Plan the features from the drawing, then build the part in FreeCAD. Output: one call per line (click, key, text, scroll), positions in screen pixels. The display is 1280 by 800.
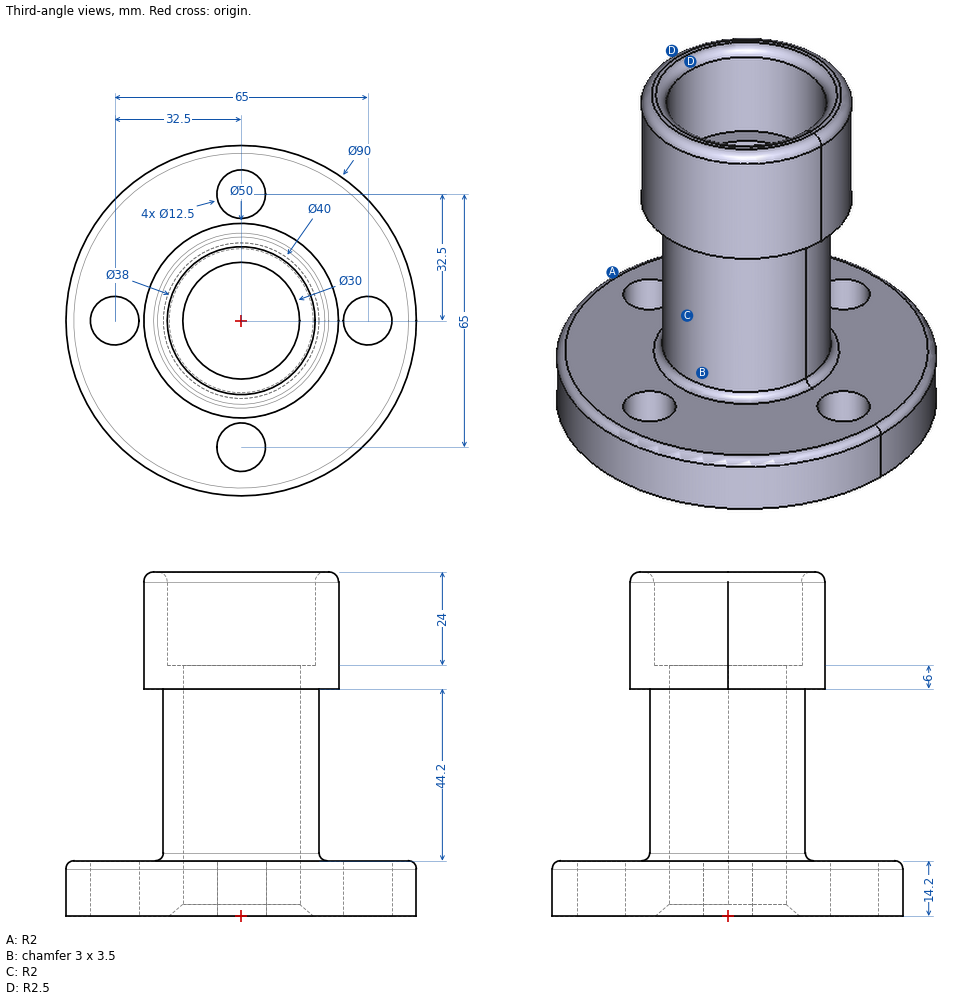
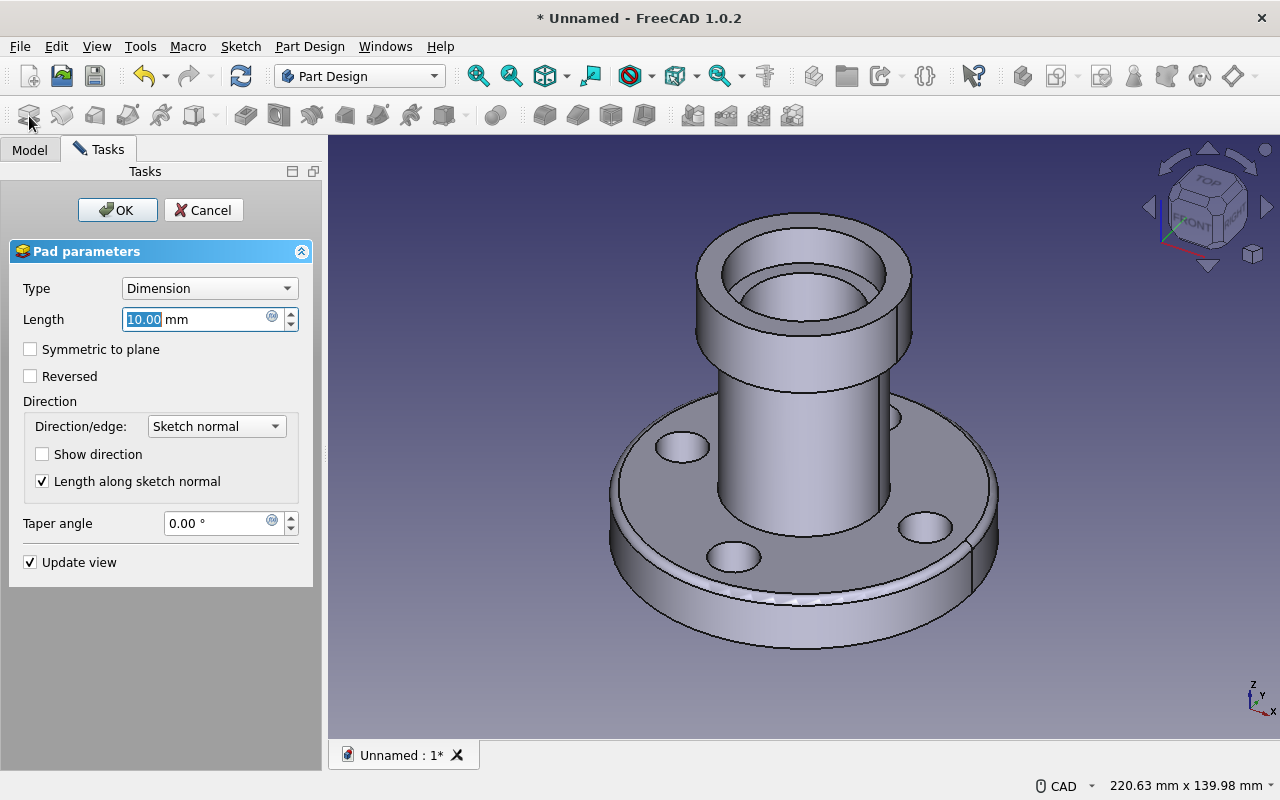
text(24)
key(Tab)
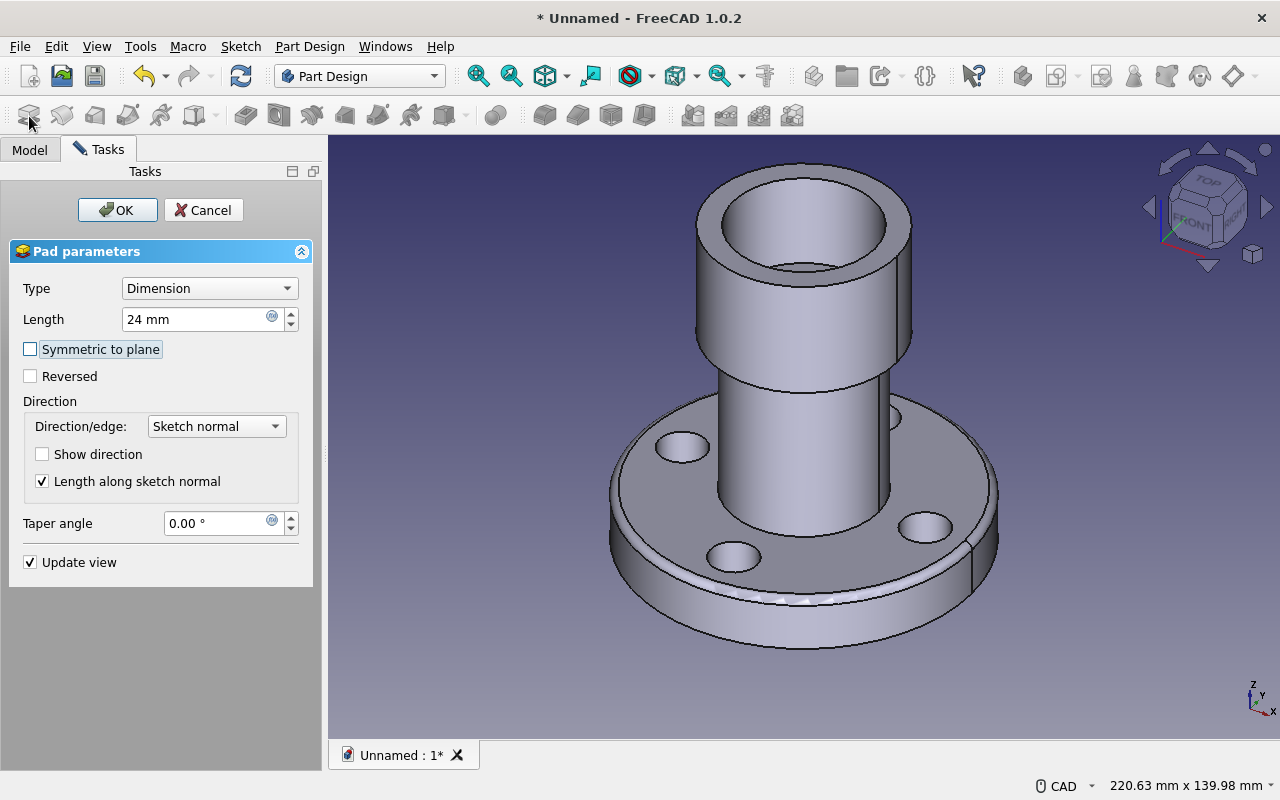
click(118, 210)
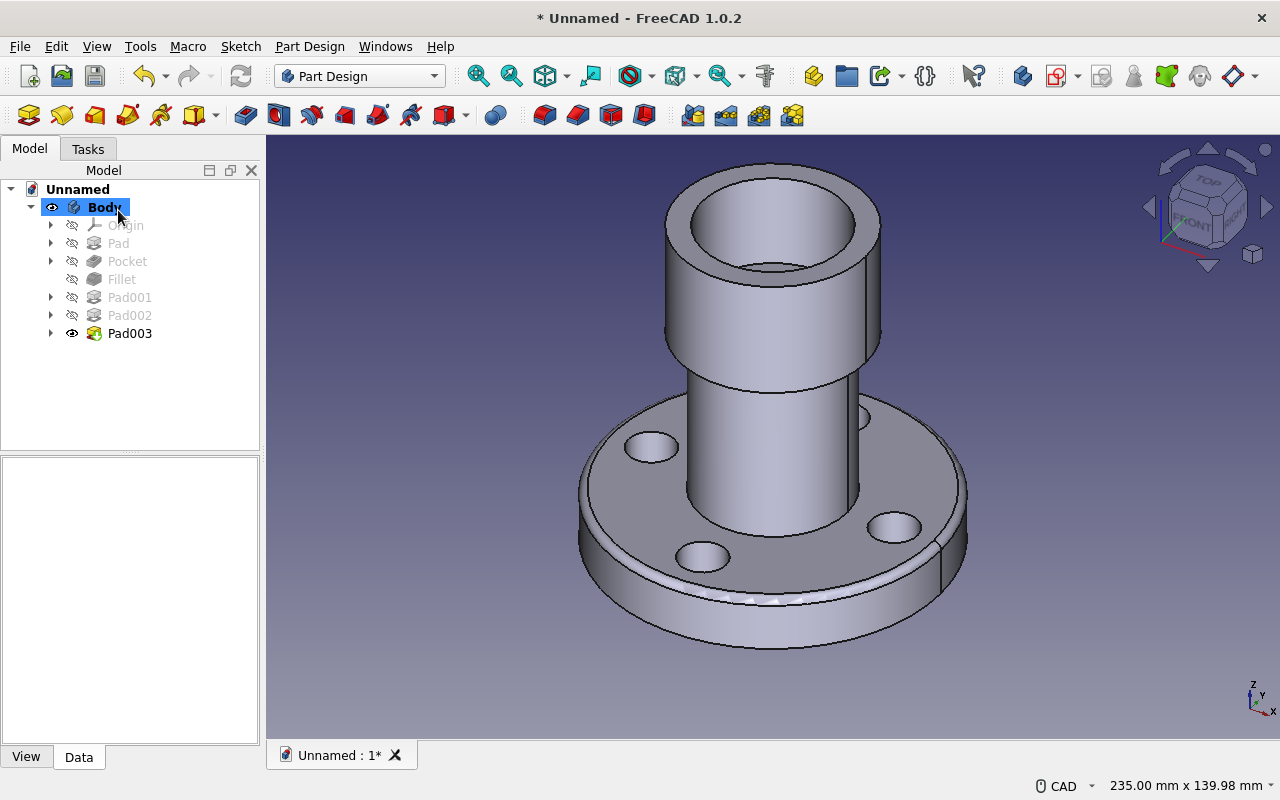
click(479, 76)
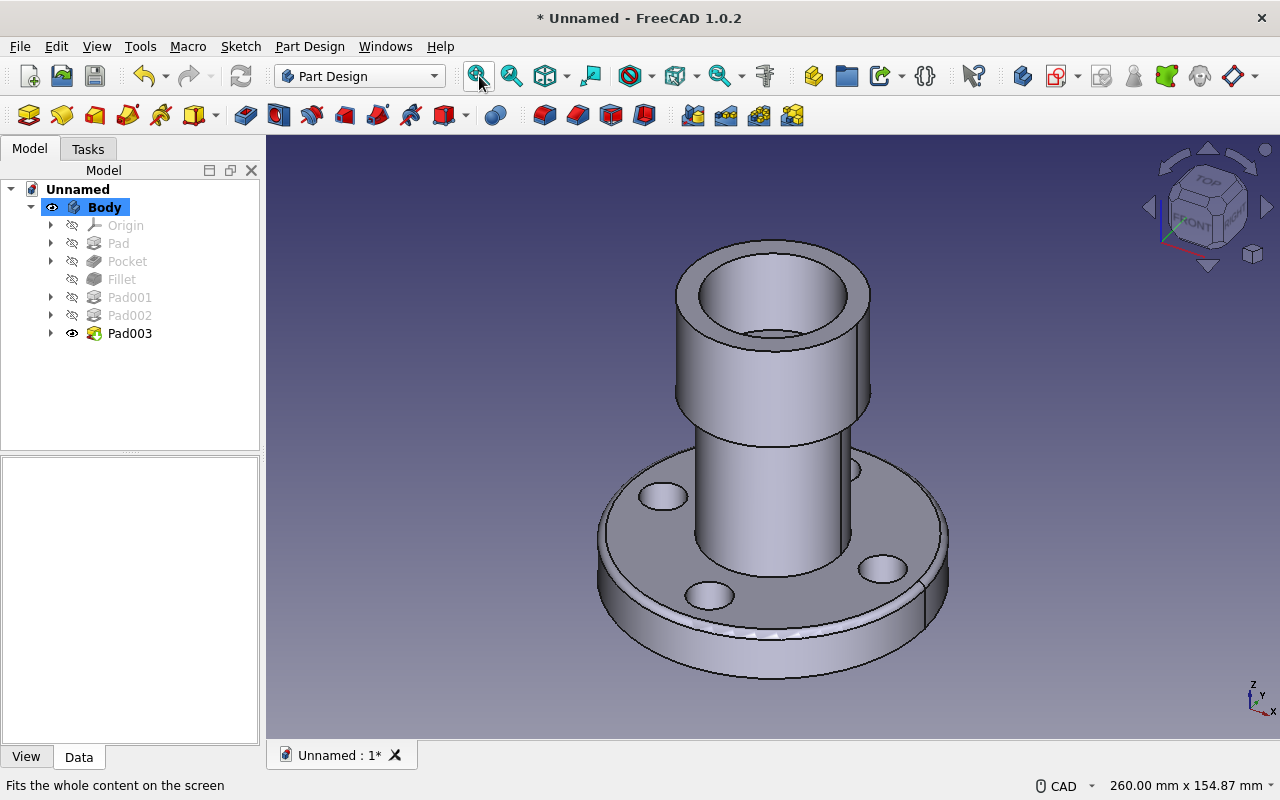
key(0)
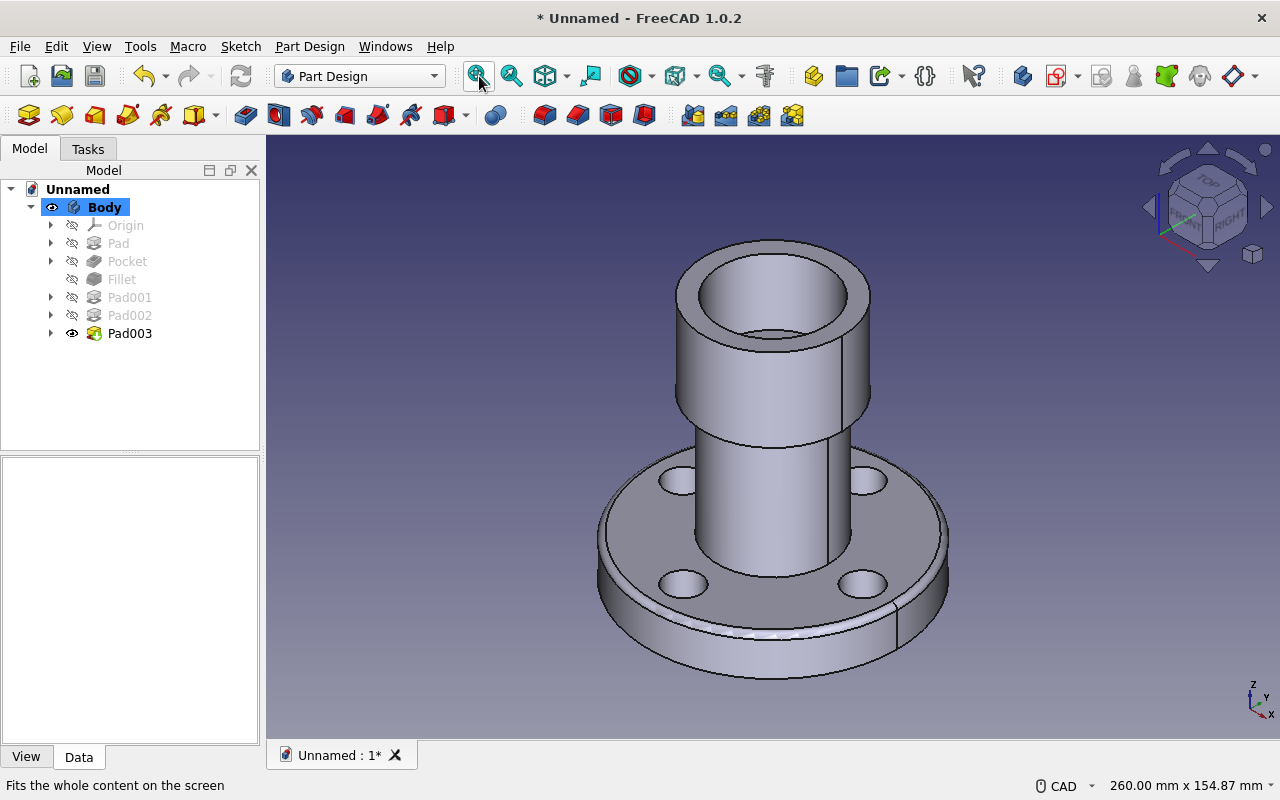
key(2)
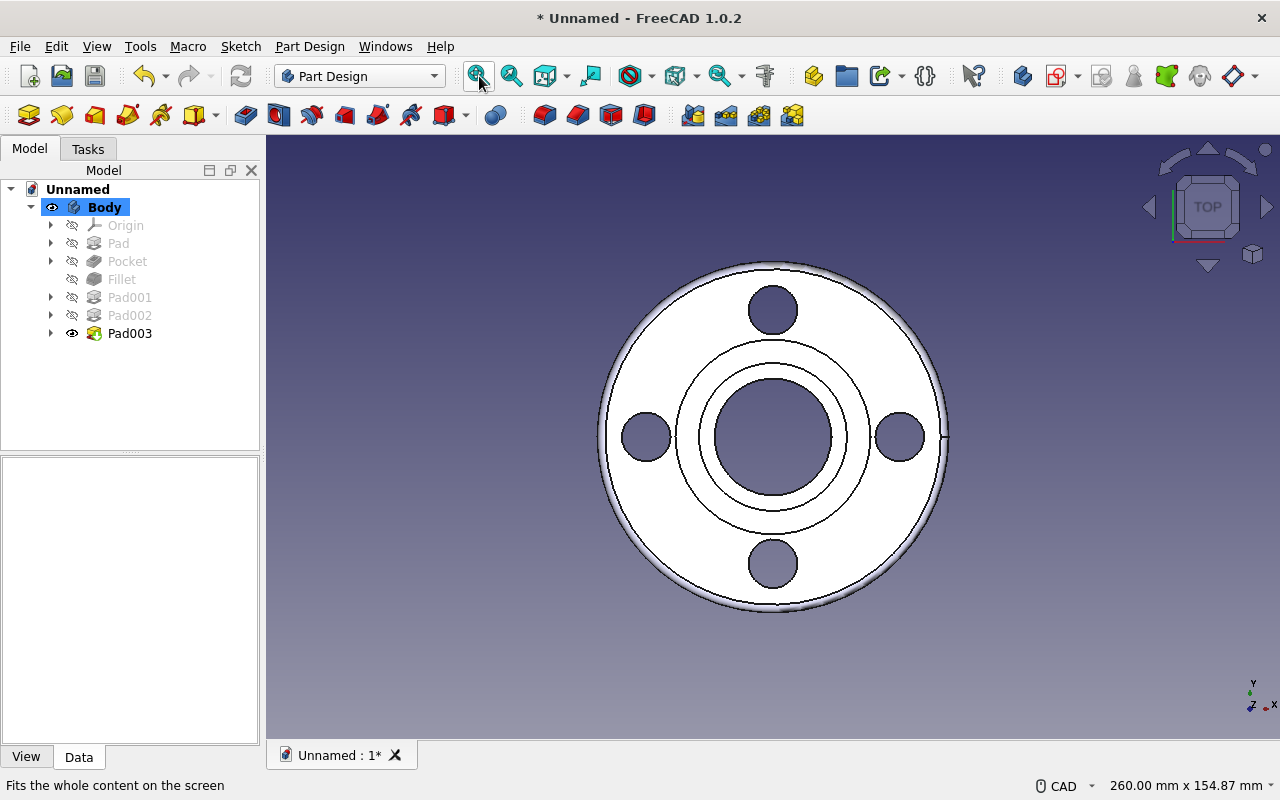
key(1)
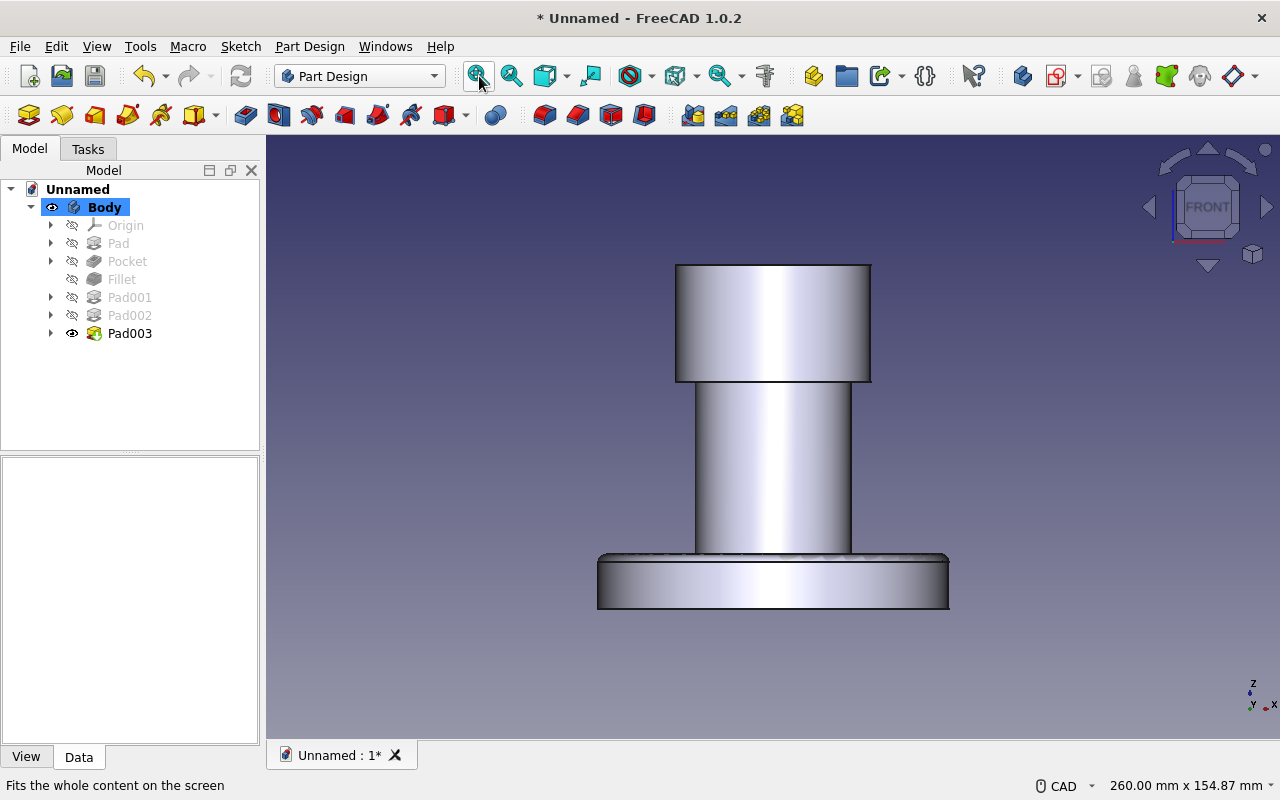
key(3)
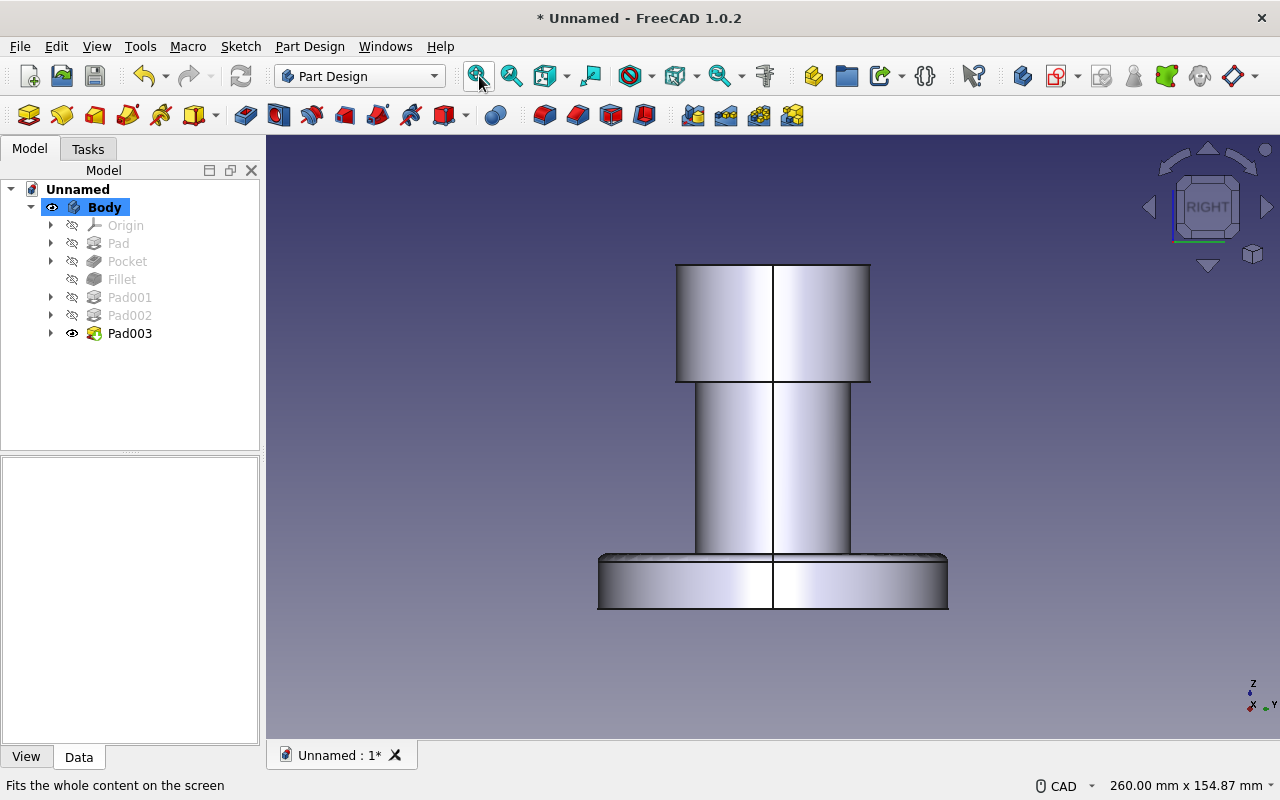
key(5)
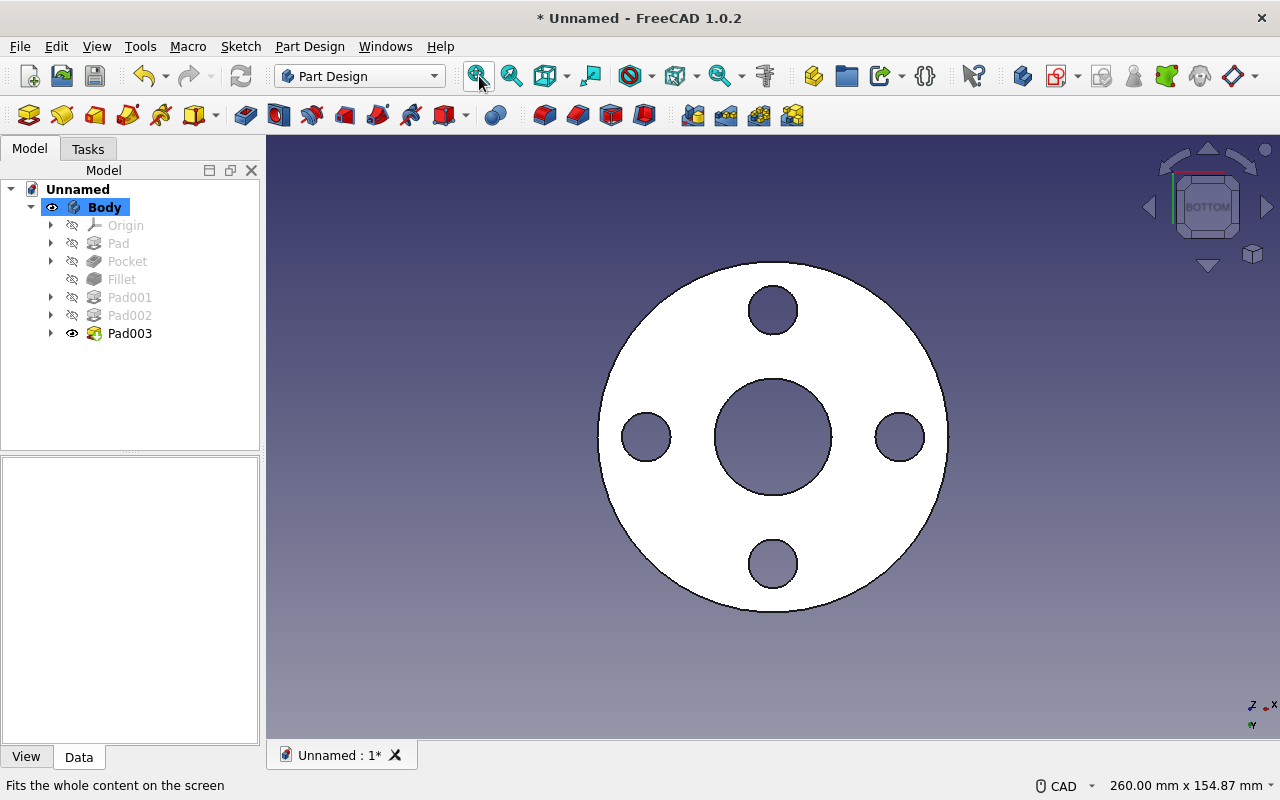
click(715, 436)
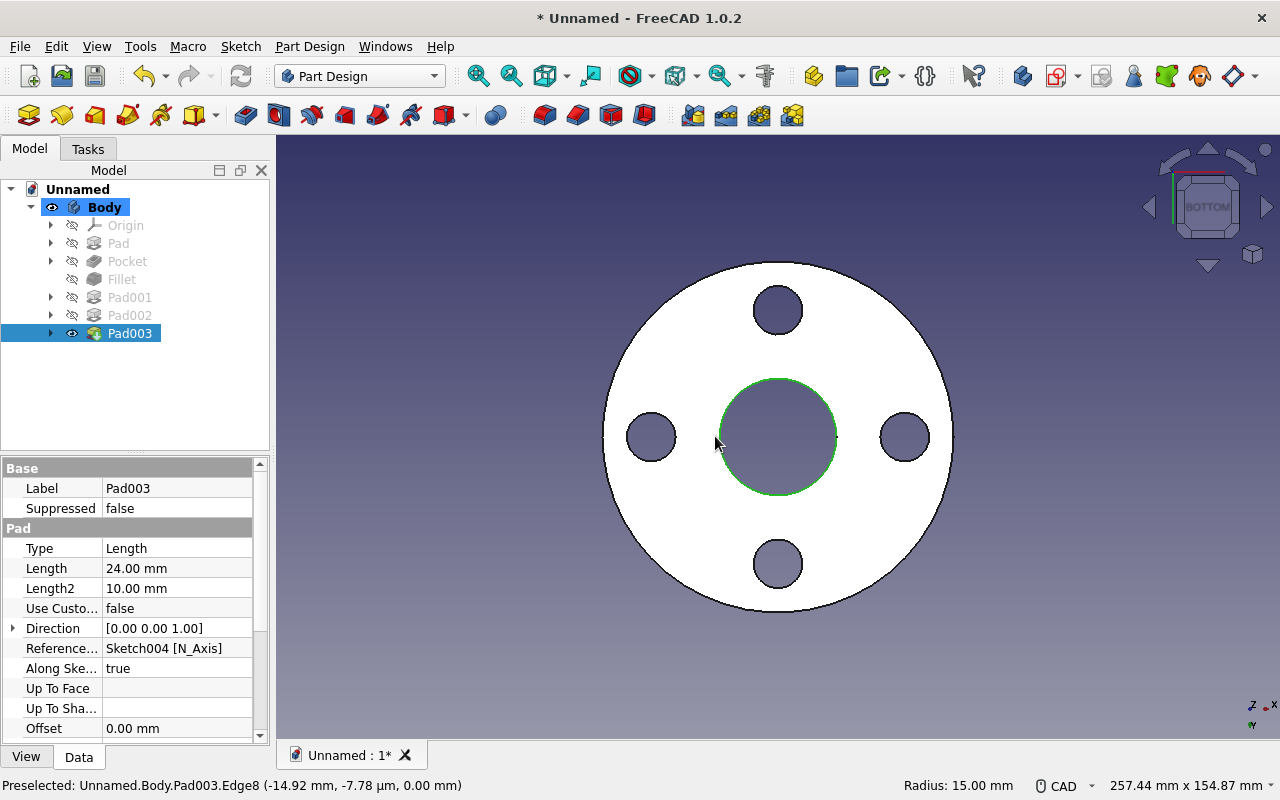
click(578, 116)